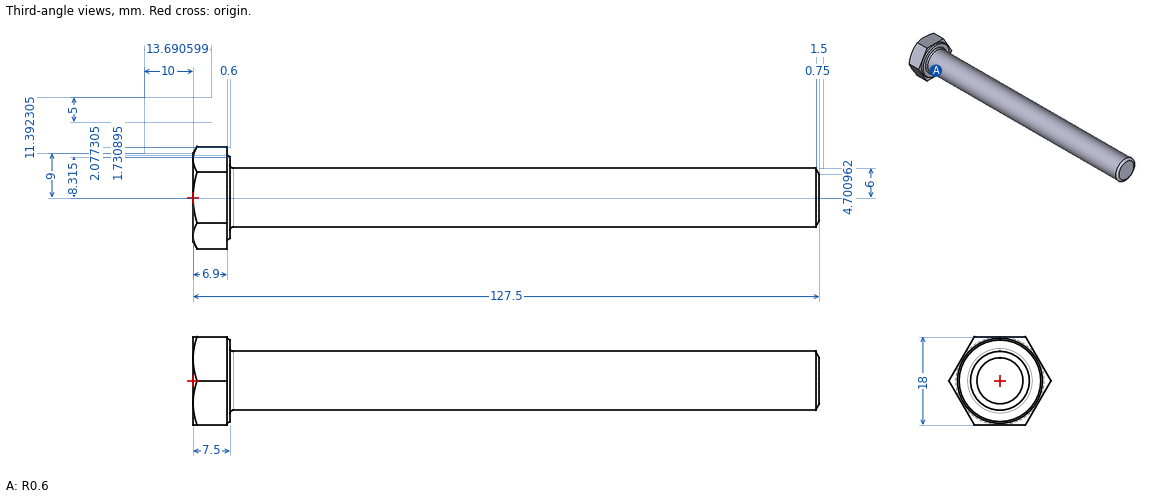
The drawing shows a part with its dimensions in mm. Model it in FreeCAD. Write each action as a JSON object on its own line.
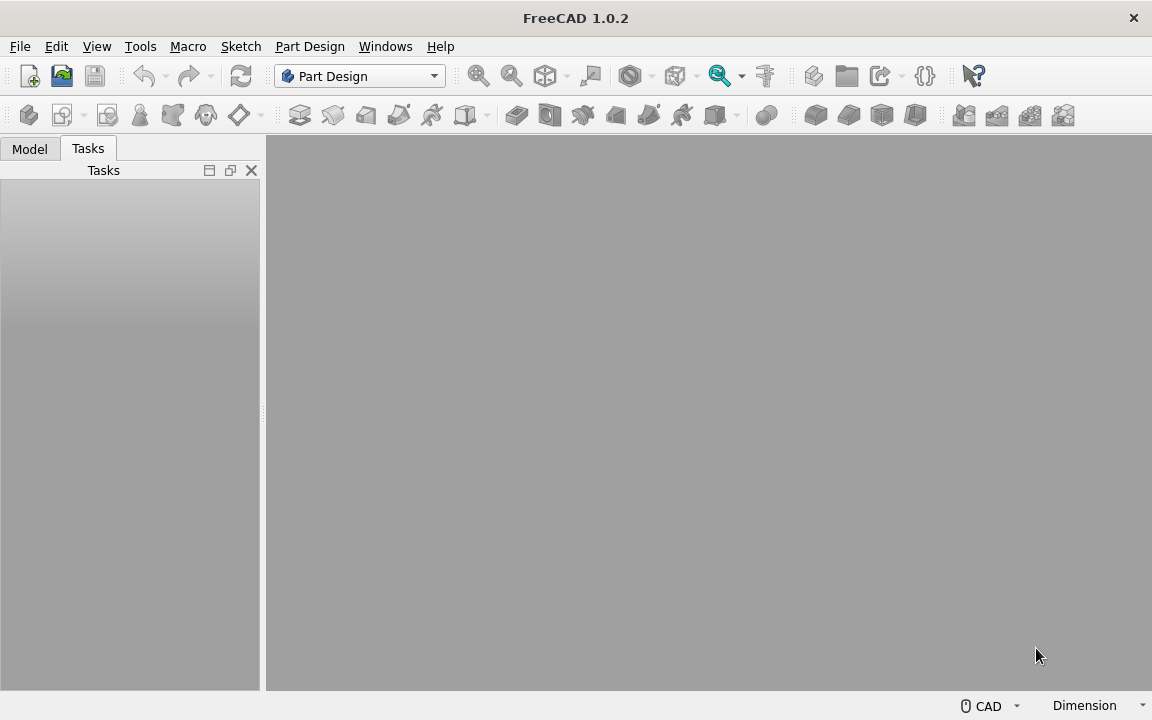
{"action": "left_click", "coordinate": [29, 76]}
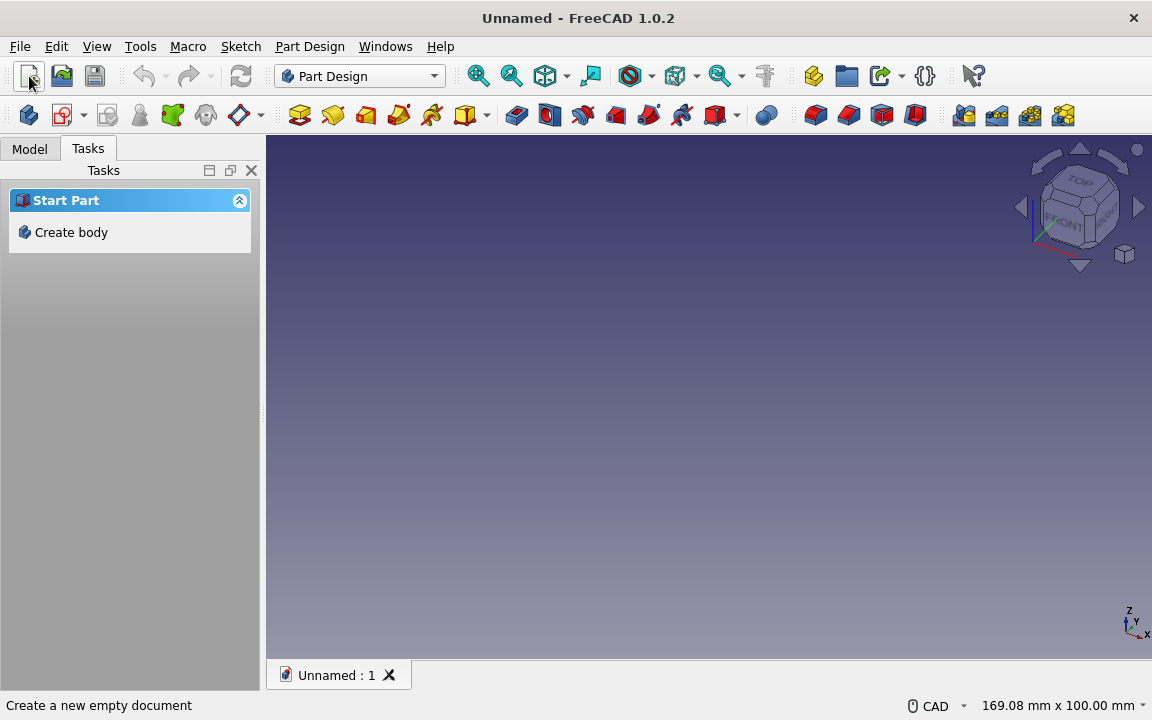
{"action": "left_click", "coordinate": [62, 116]}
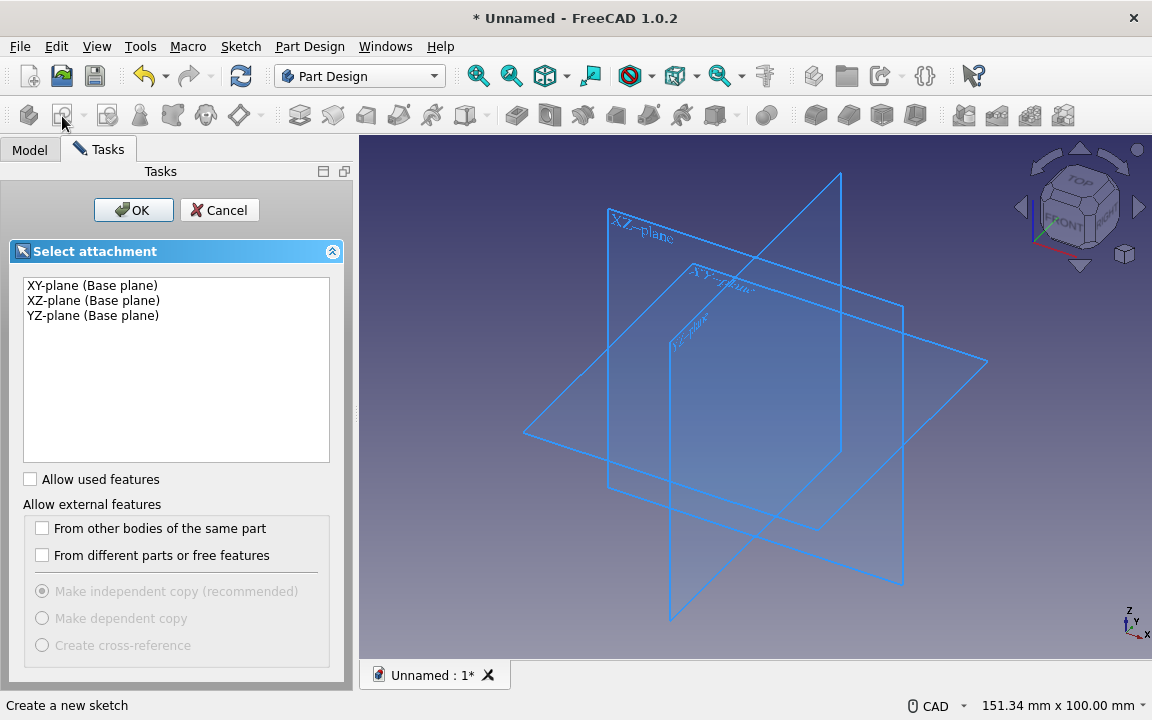
{"action": "left_click", "coordinate": [84, 316]}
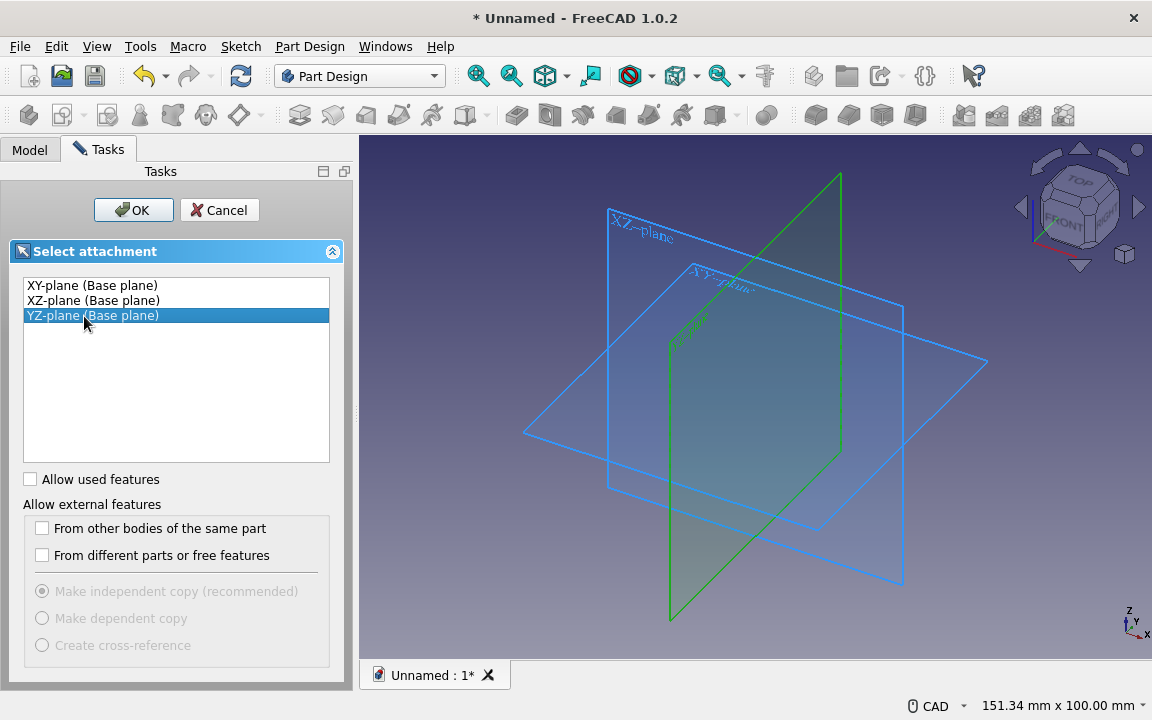
{"action": "left_click", "coordinate": [134, 210]}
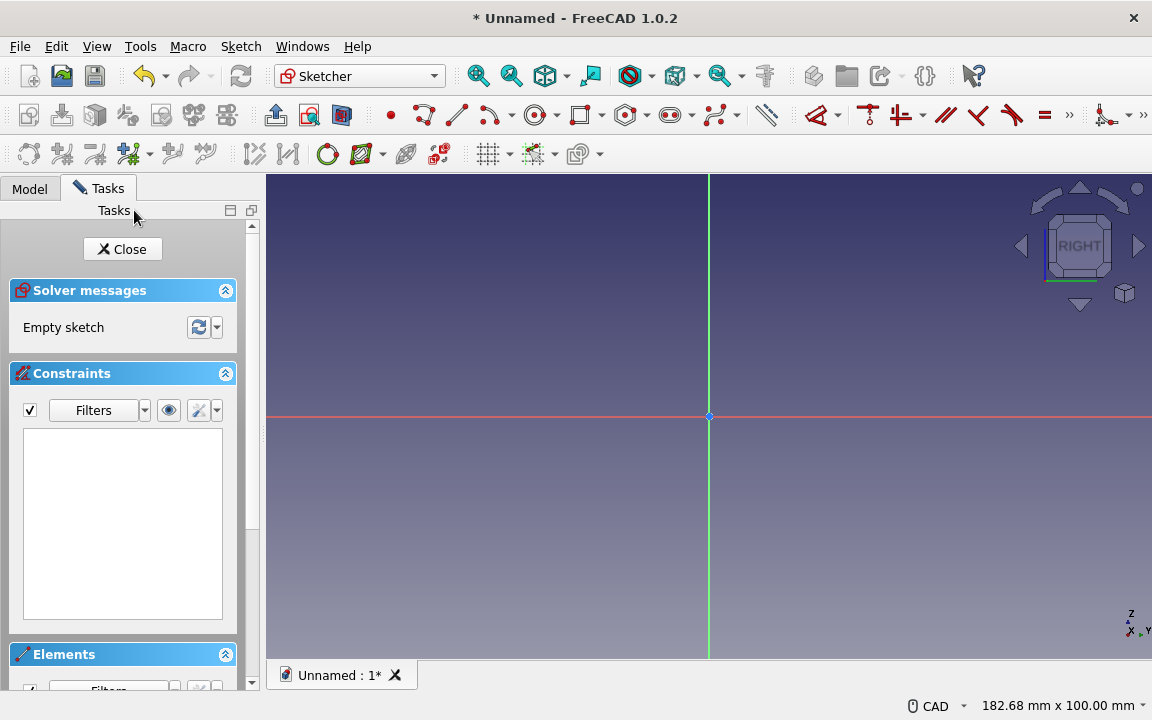
{"action": "scroll", "coordinate": [739, 416], "scroll_direction": "up", "scroll_amount": 6}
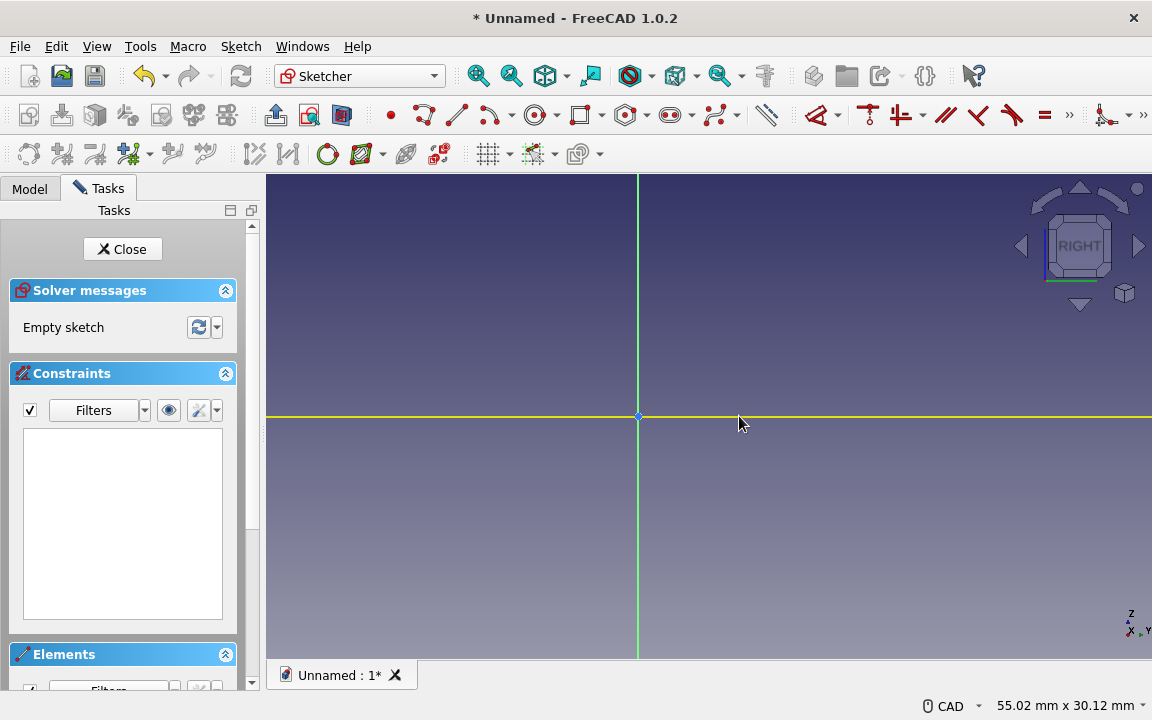
{"action": "left_click", "coordinate": [624, 116]}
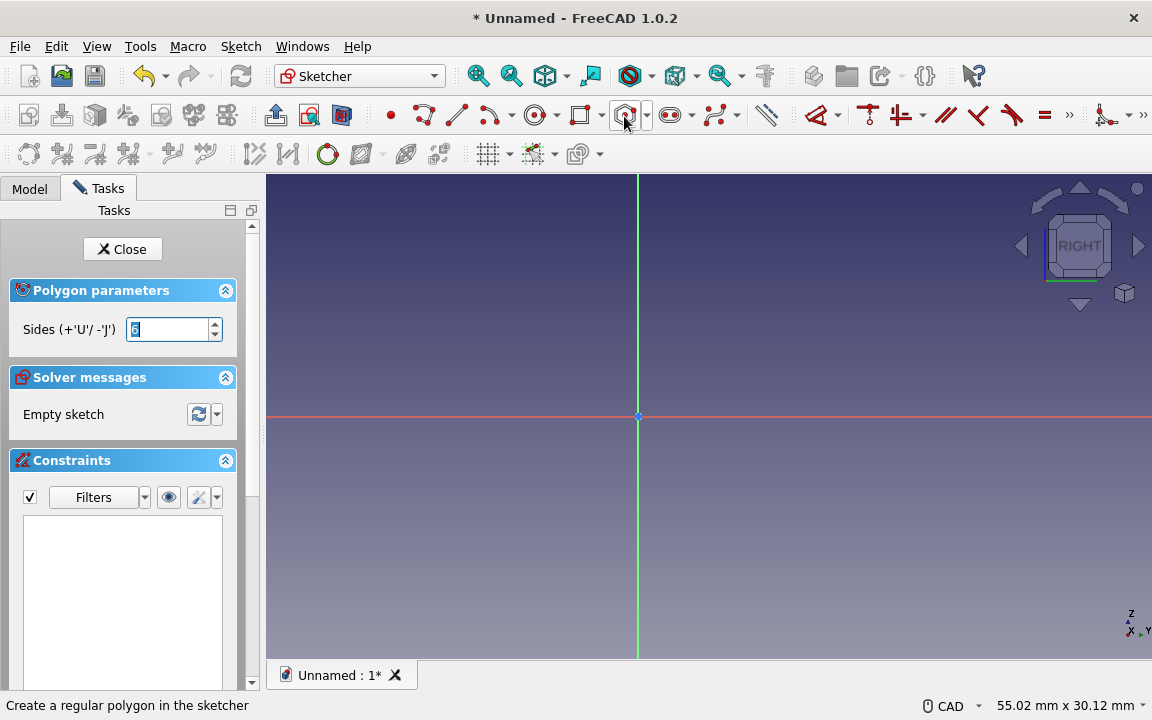
{"action": "left_click", "coordinate": [638, 416]}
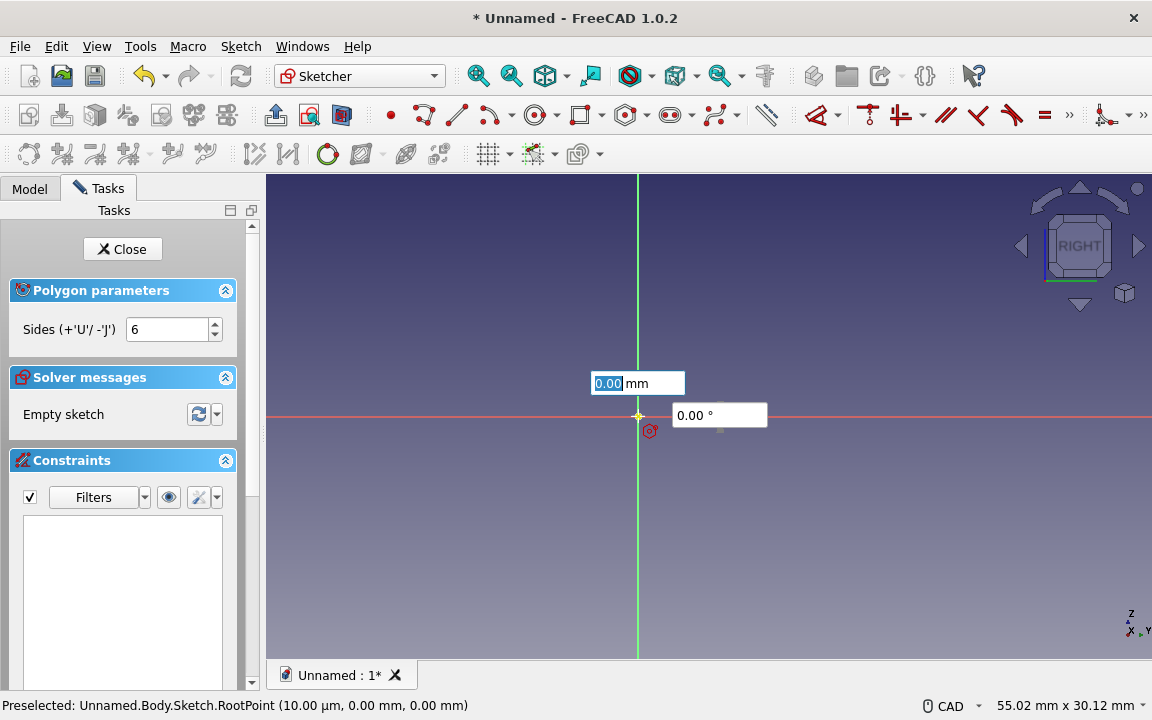
{"action": "left_click", "coordinate": [805, 416]}
{"action": "right_click", "coordinate": [805, 416]}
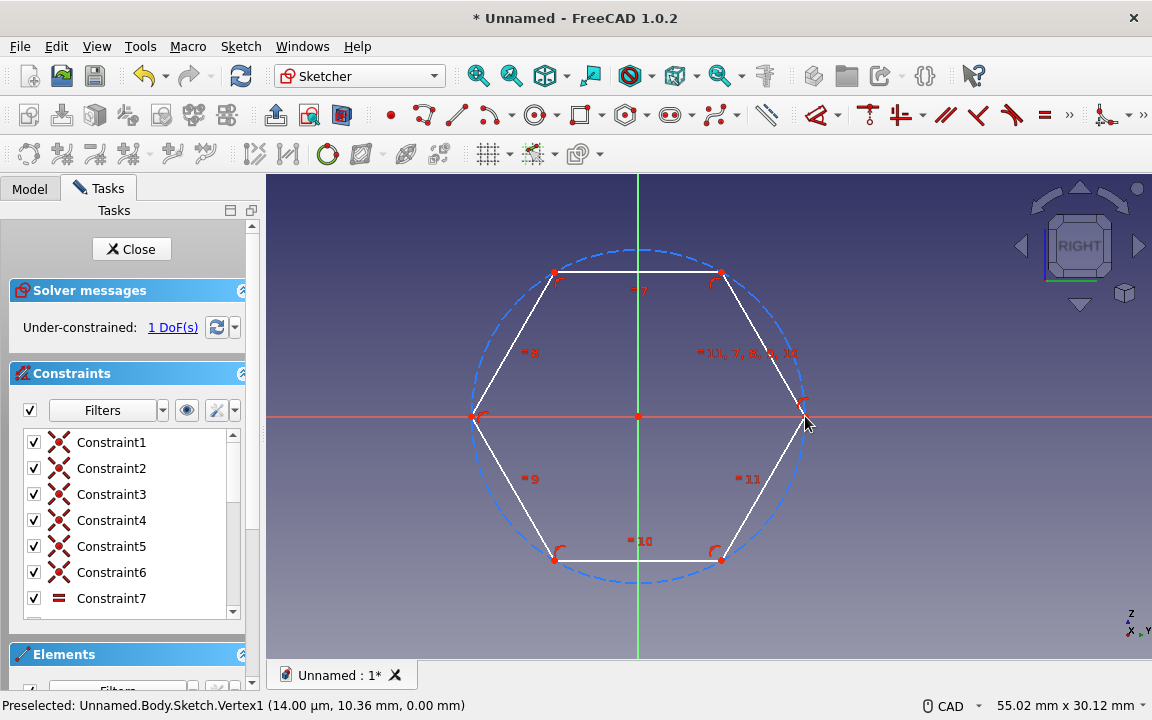
{"action": "left_click", "coordinate": [816, 116]}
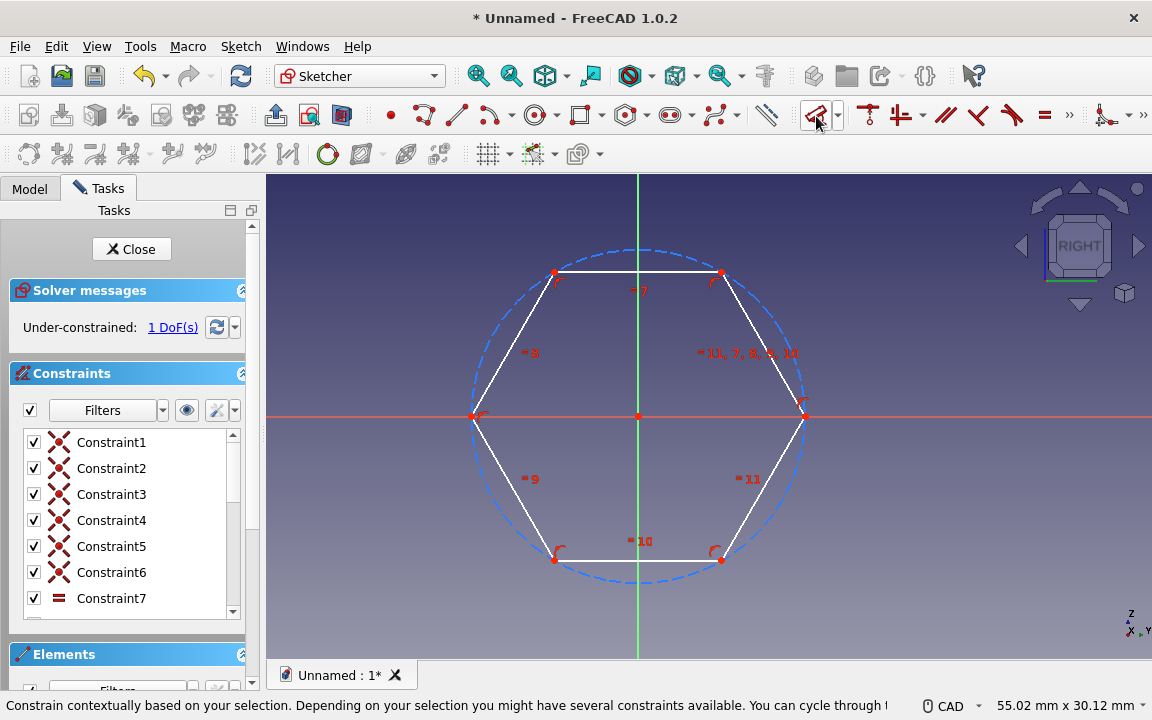
{"action": "left_click", "coordinate": [555, 561]}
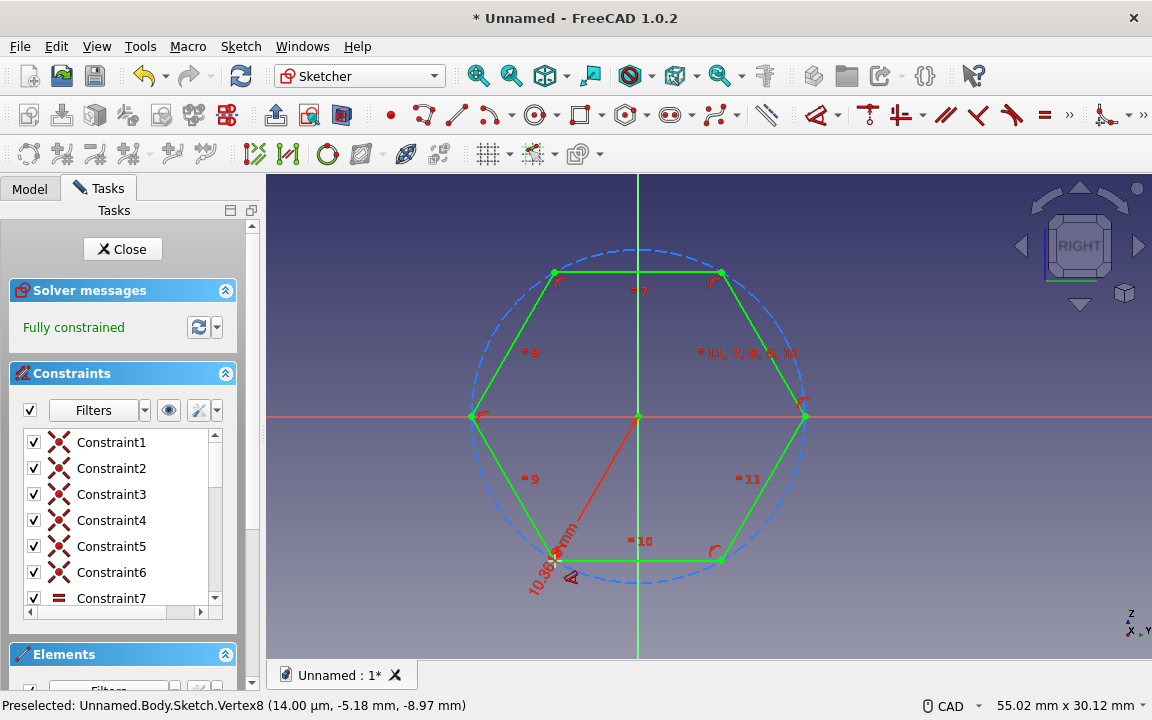
{"action": "left_click", "coordinate": [722, 272]}
{"action": "left_click", "coordinate": [804, 315]}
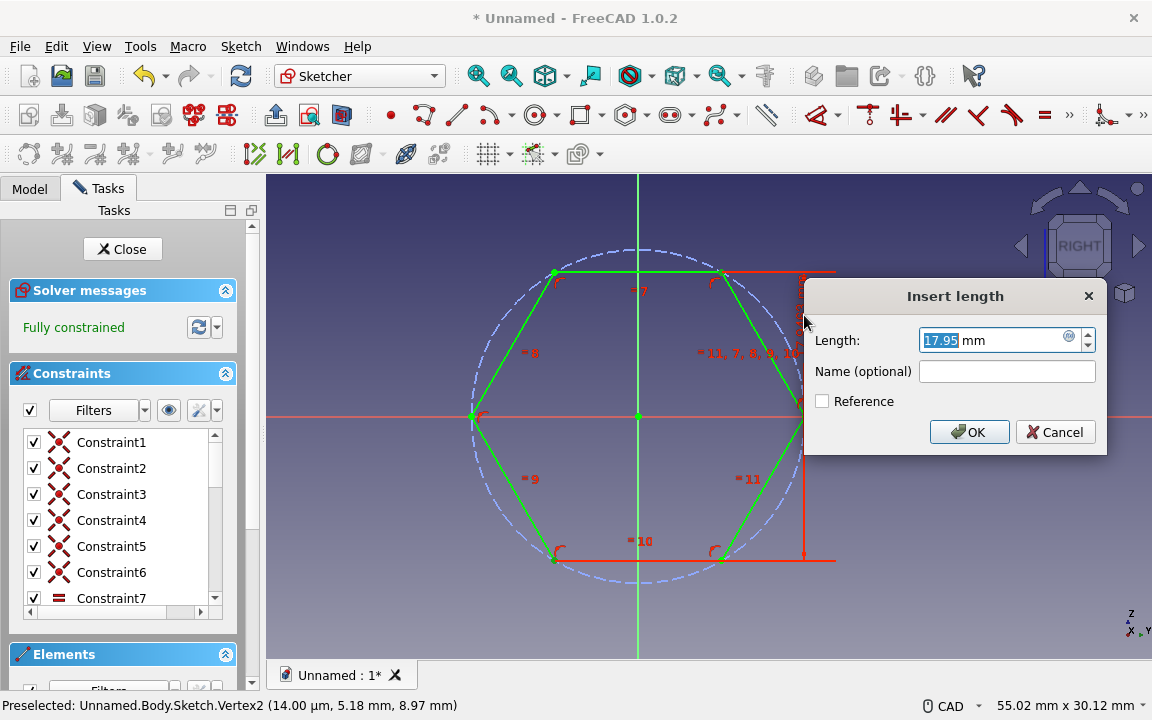
{"action": "type", "text": "18"}
{"action": "key", "text": "Return"}
{"action": "key", "text": "Escape"}